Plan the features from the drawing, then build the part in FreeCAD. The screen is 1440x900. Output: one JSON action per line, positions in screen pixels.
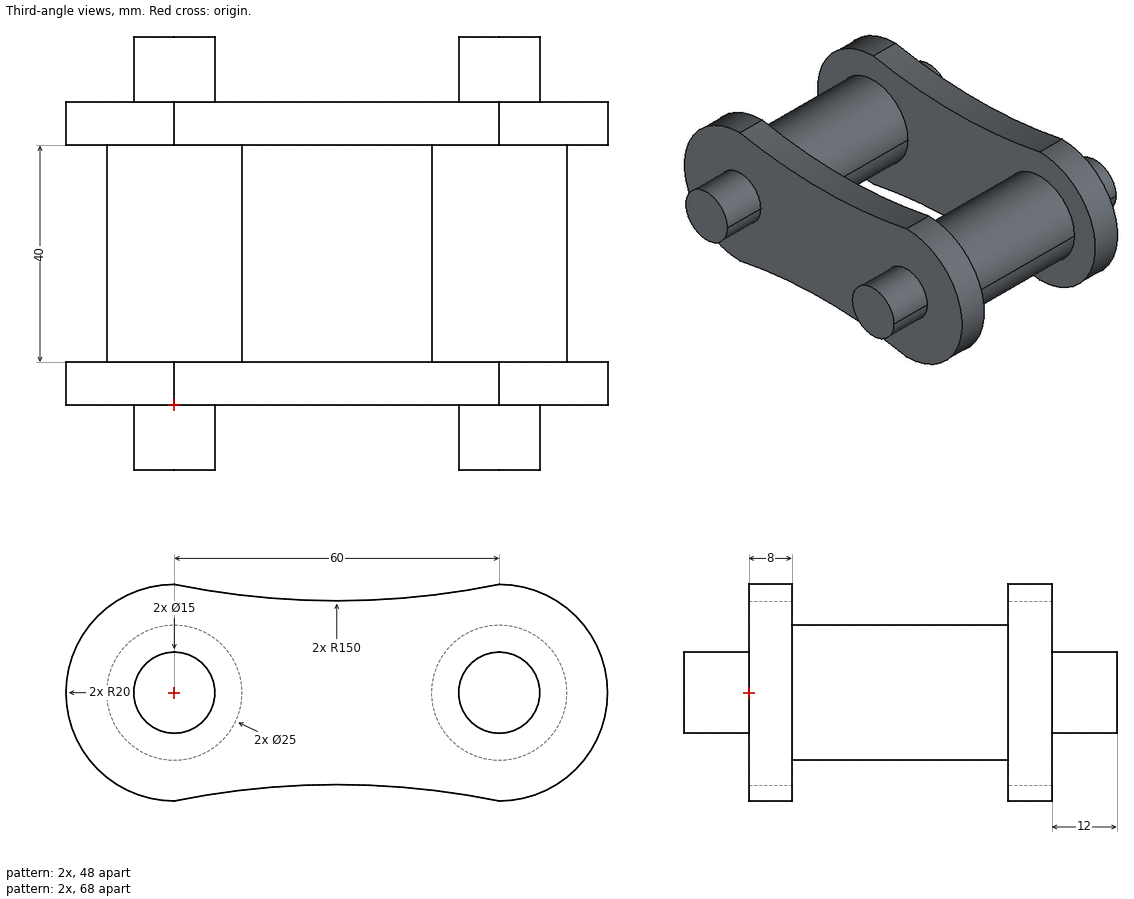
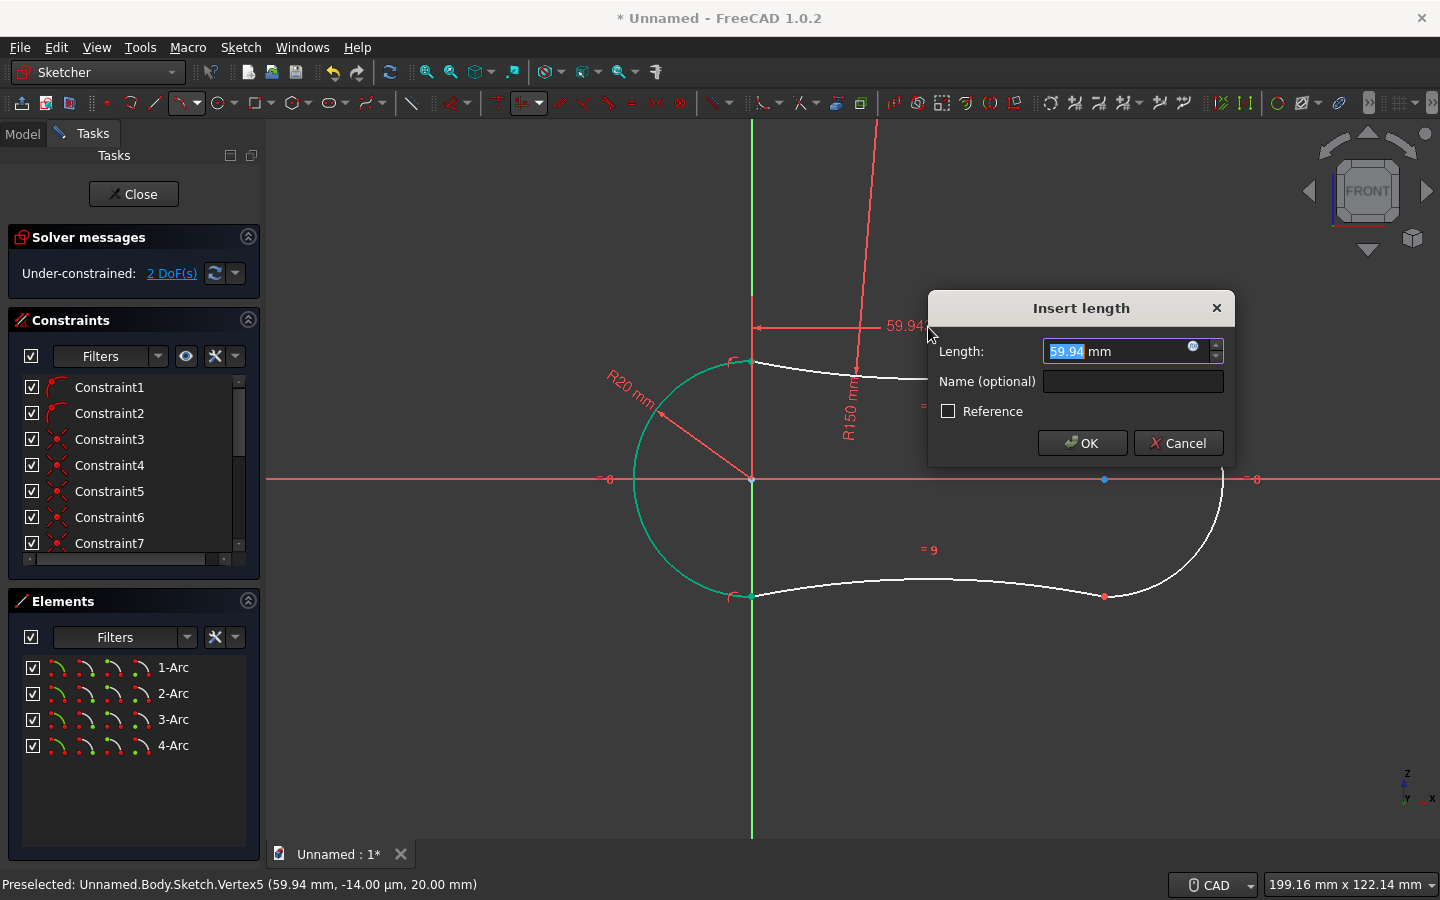
{"action": "type", "text": "60"}
{"action": "key", "text": "Return"}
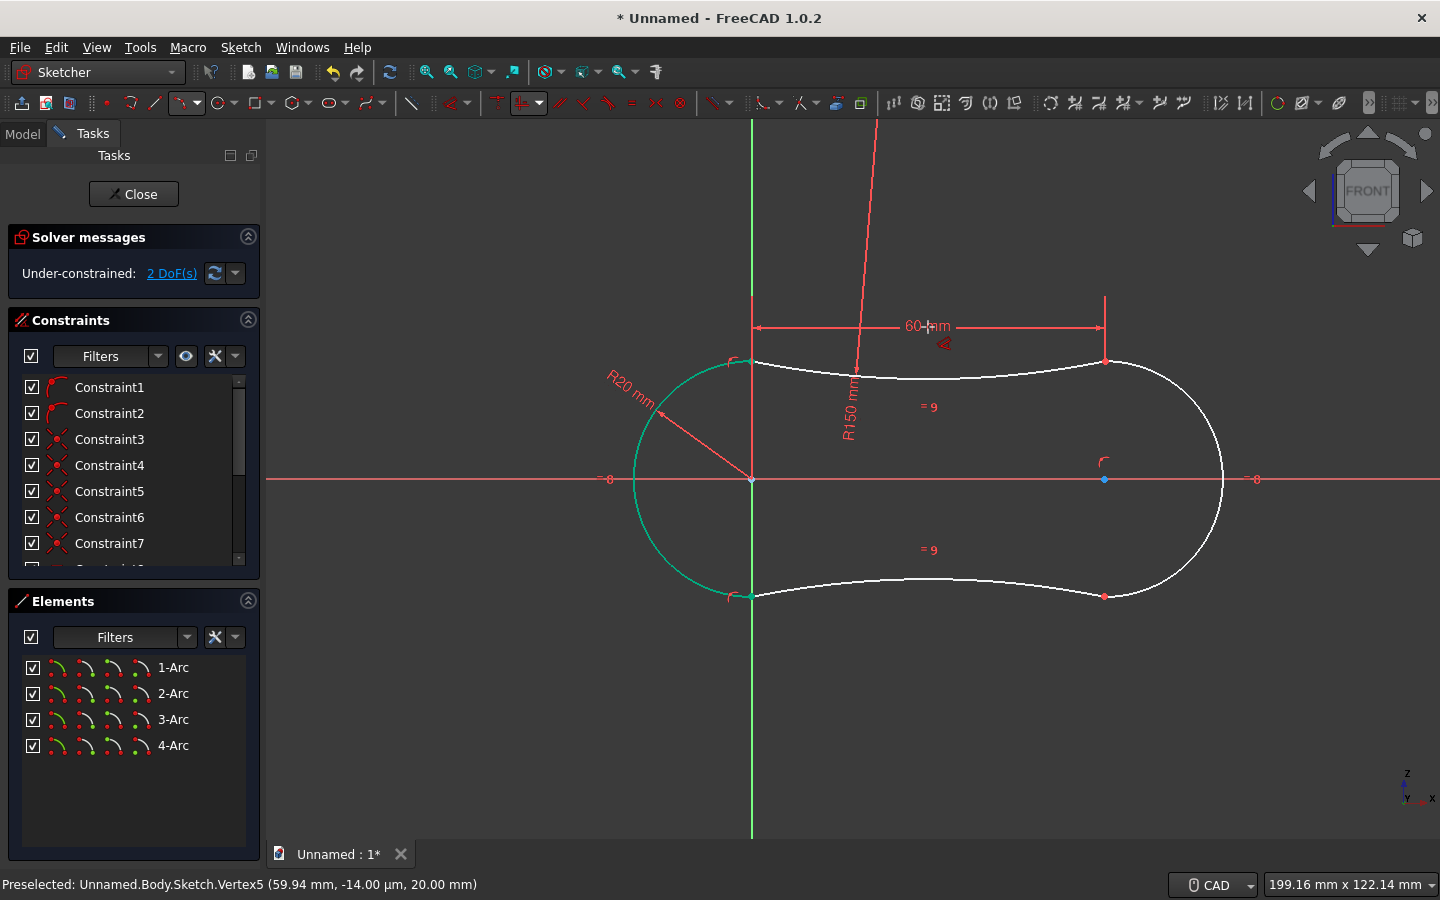
{"action": "left_click", "coordinate": [1105, 597]}
{"action": "left_click", "coordinate": [928, 631]}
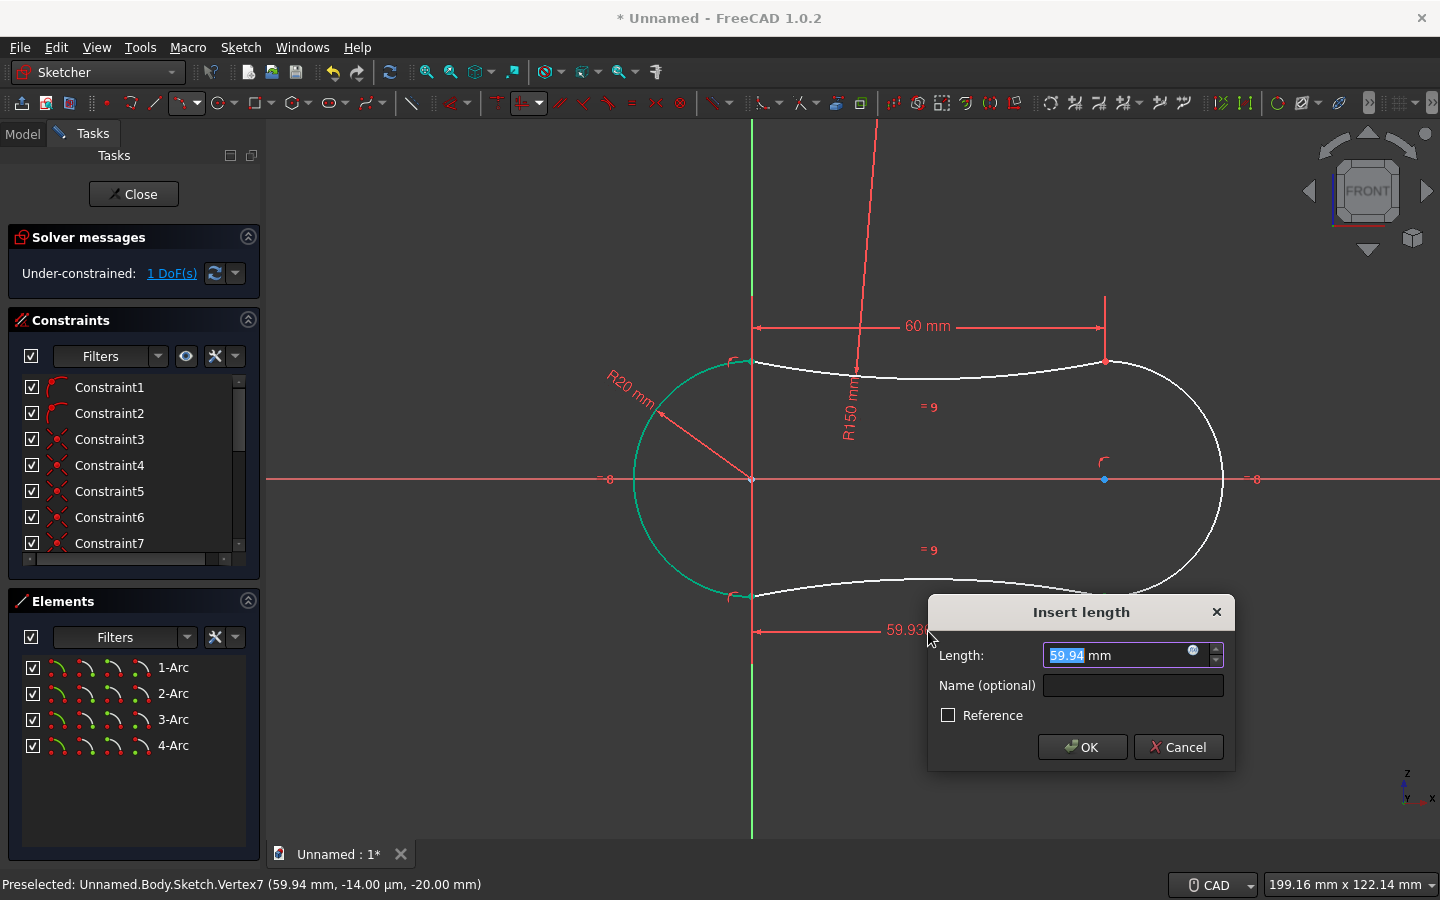
{"action": "type", "text": "60"}
{"action": "key", "text": "Return"}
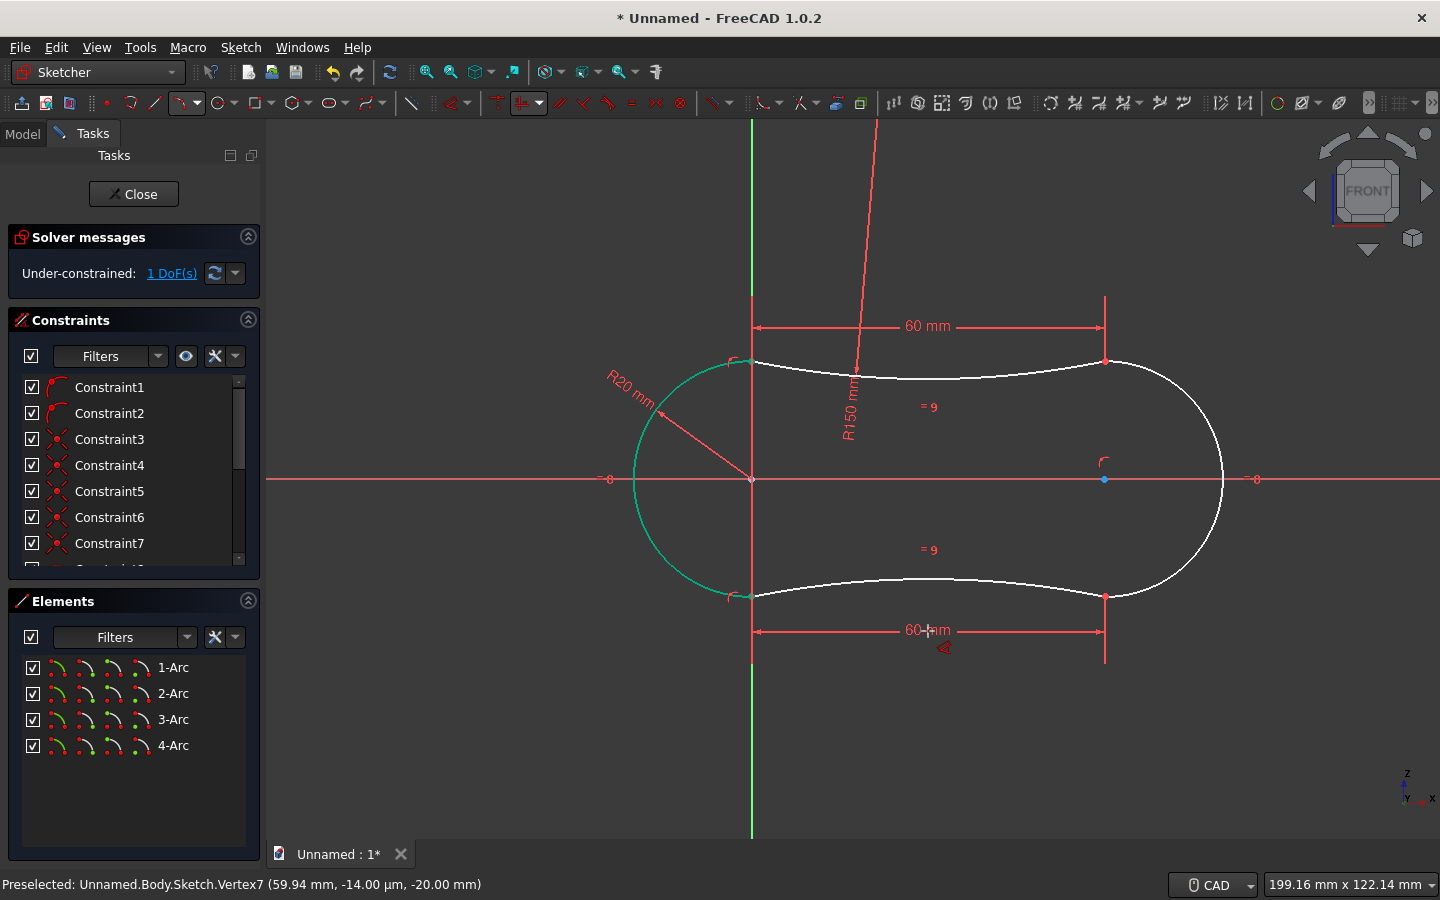
{"action": "left_click", "coordinate": [1105, 479]}
{"action": "left_click", "coordinate": [928, 513]}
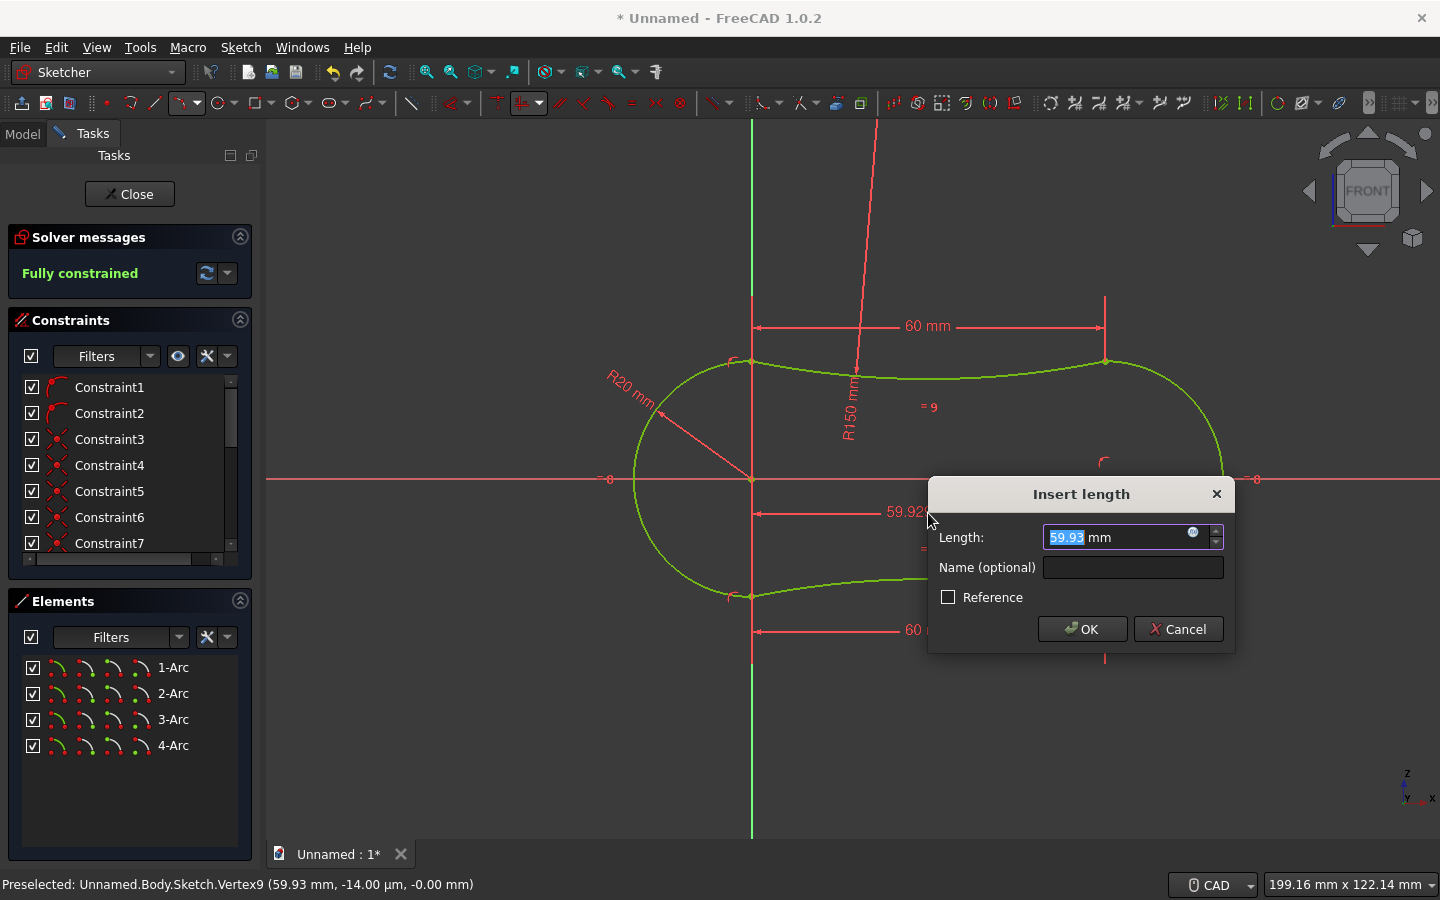
{"action": "type", "text": "60"}
{"action": "key", "text": "Return"}
{"action": "key", "text": "Escape"}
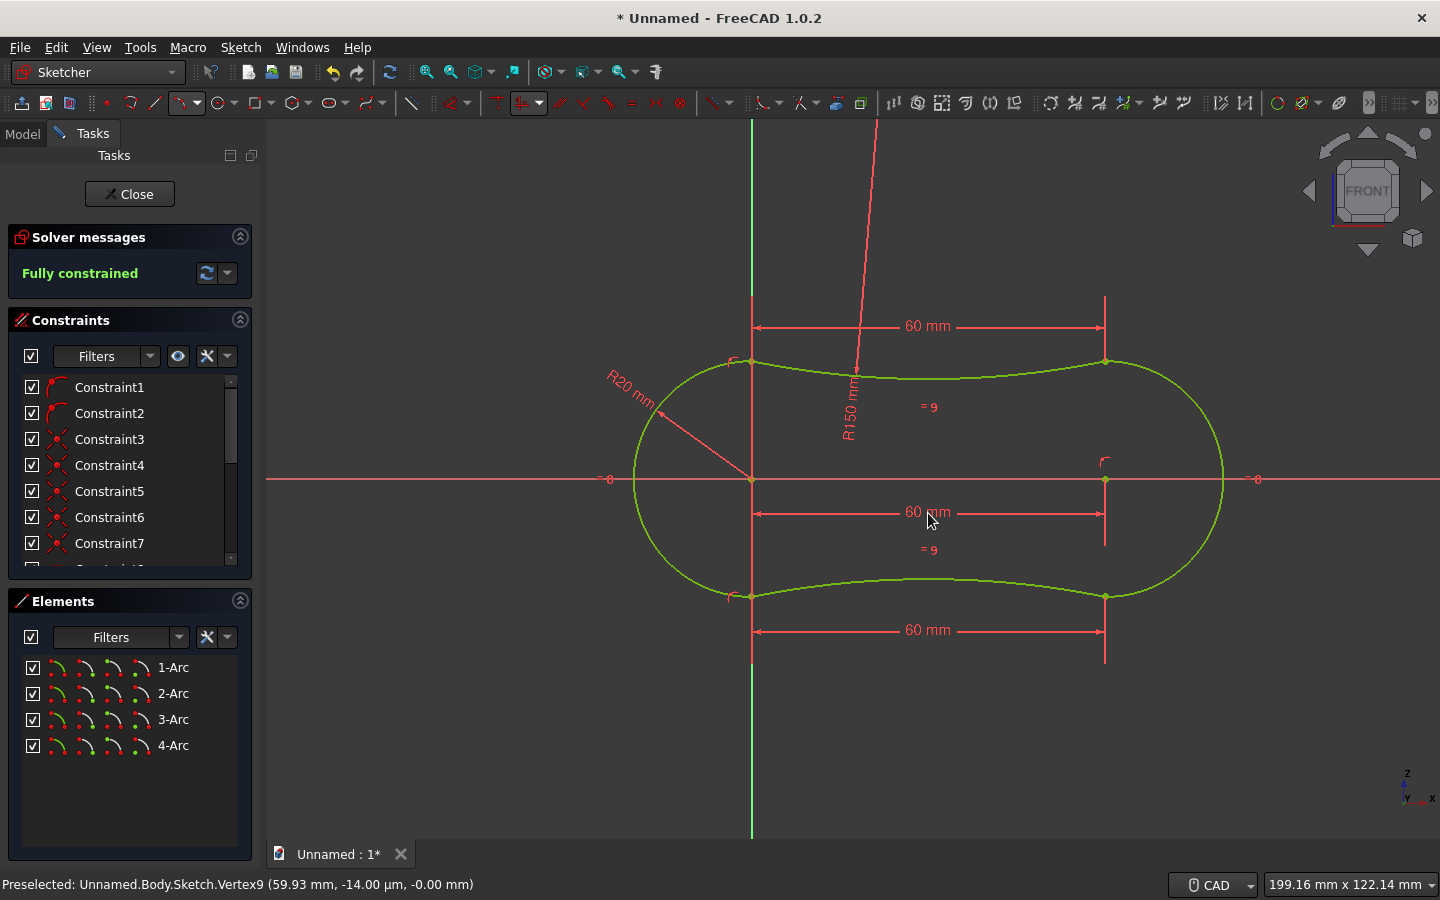
{"action": "left_click", "coordinate": [130, 194]}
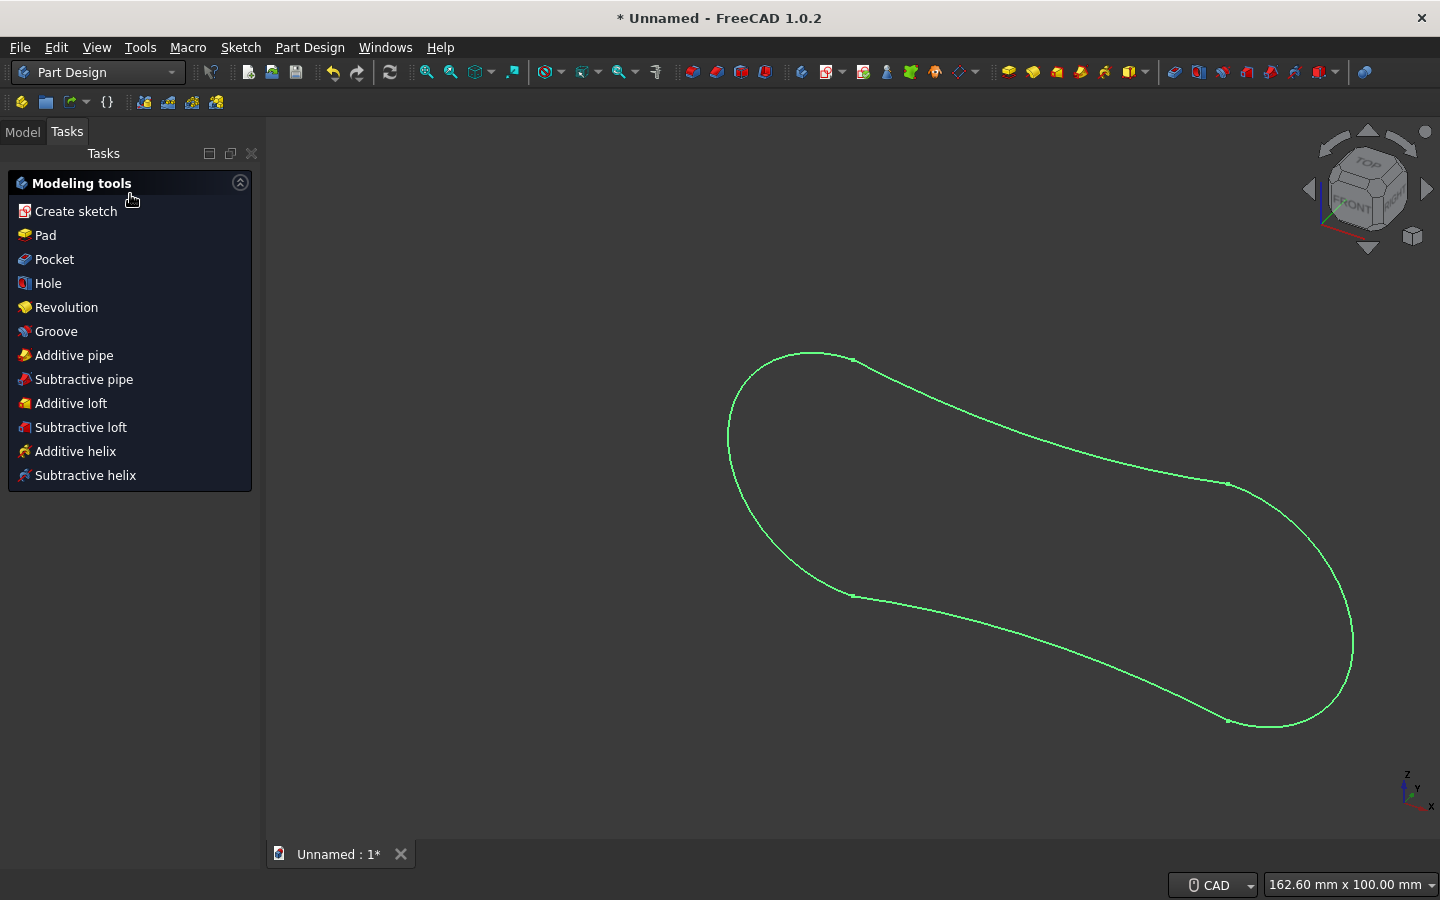
{"action": "left_click", "coordinate": [1010, 72]}